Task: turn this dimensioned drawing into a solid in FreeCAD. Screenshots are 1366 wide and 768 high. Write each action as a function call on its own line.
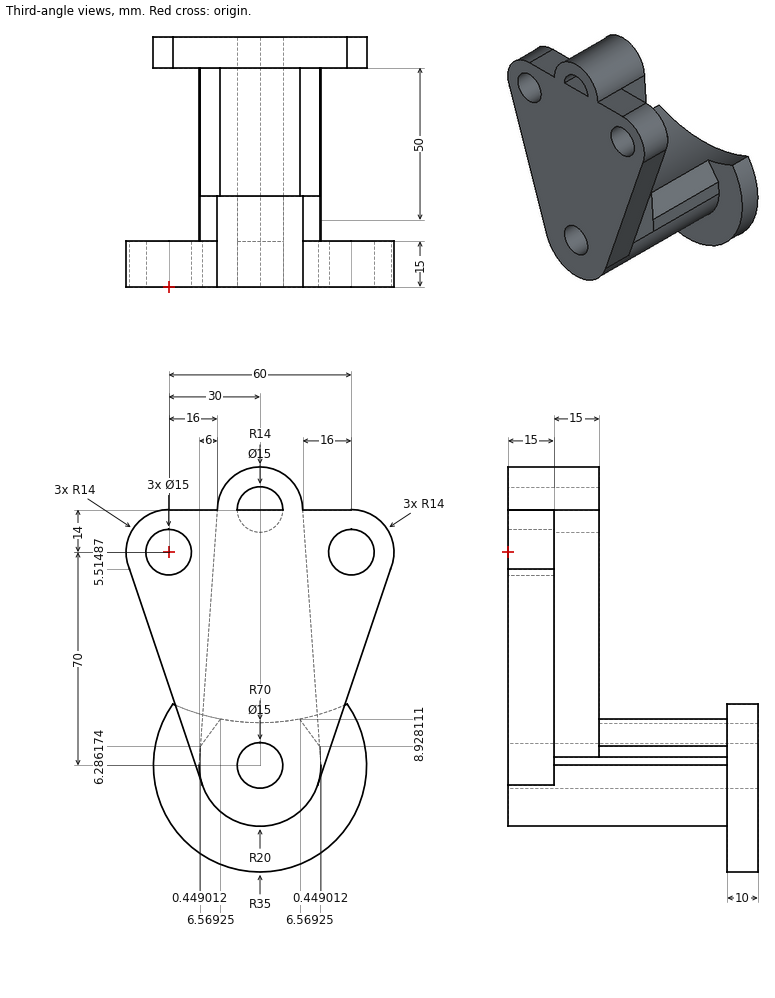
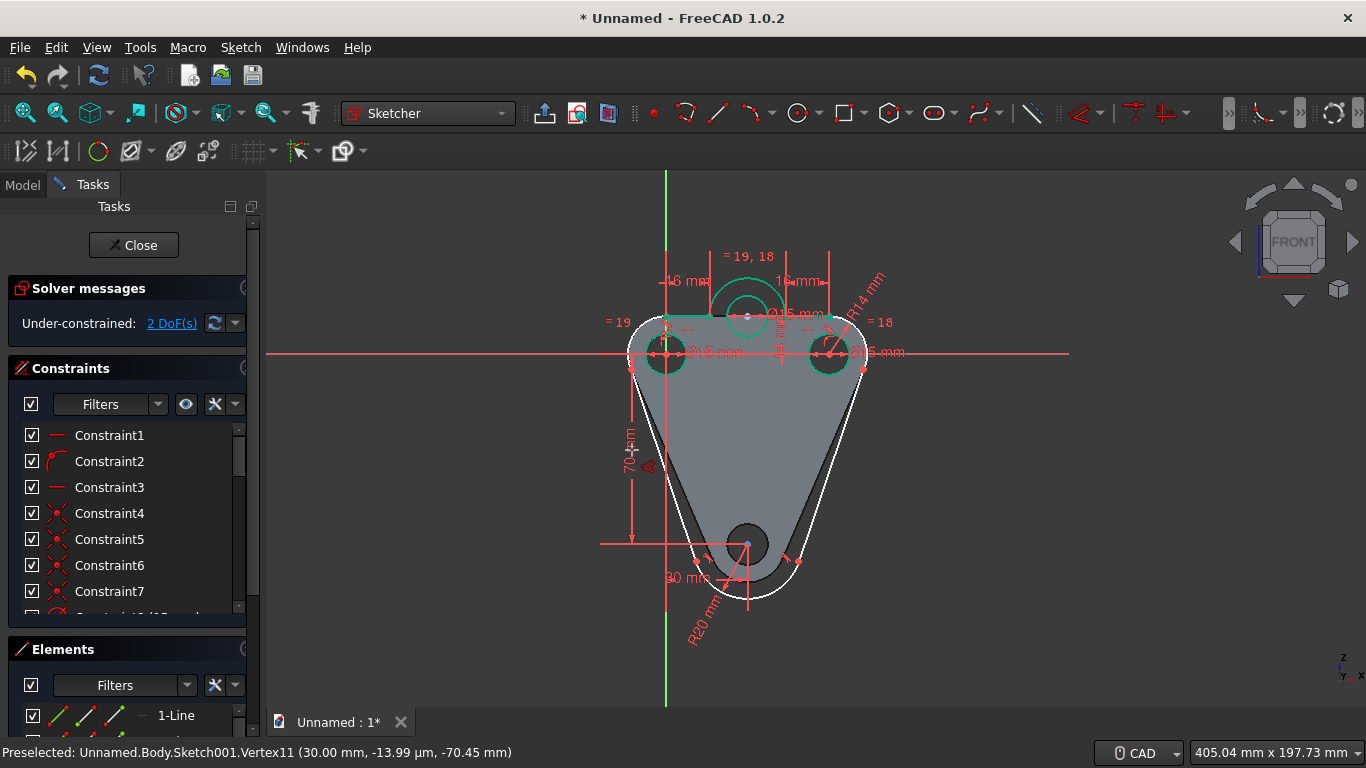
scroll(631, 370, up, 5)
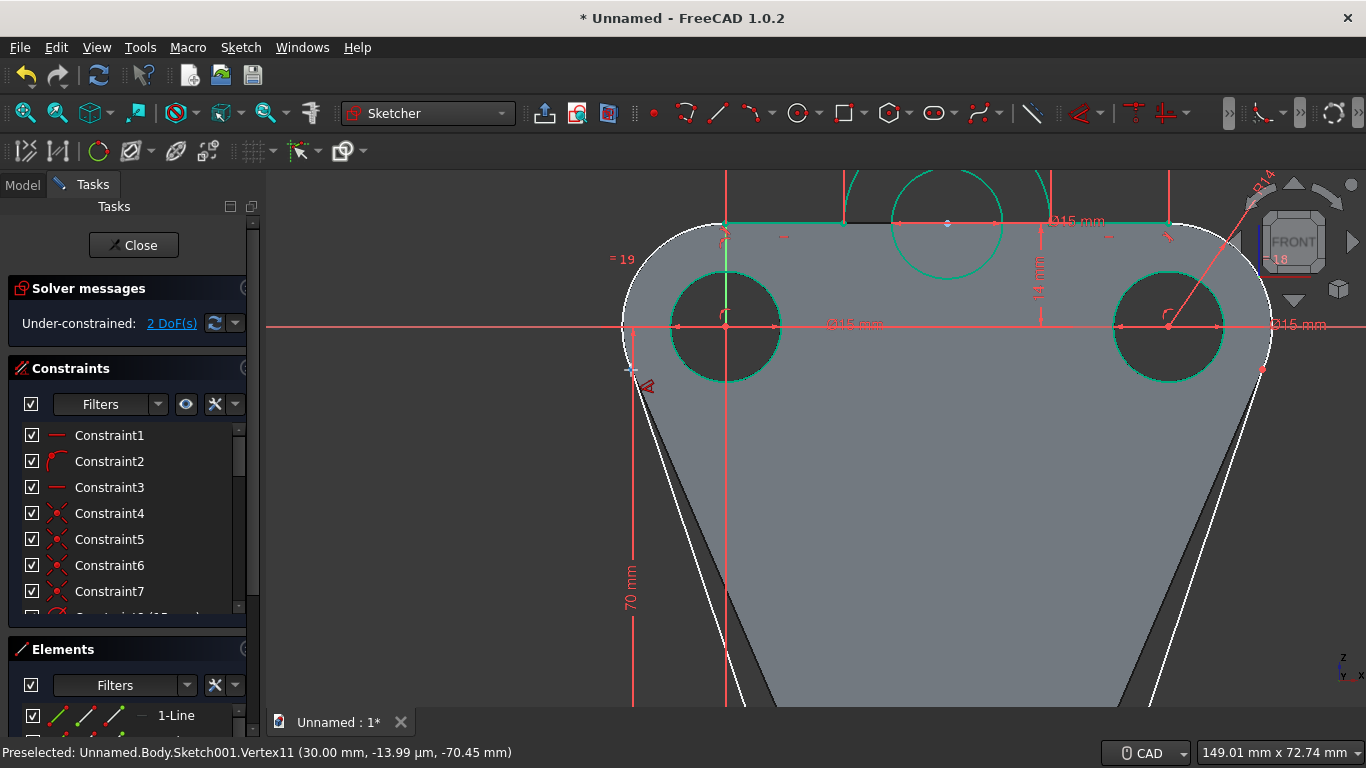
click(632, 369)
click(598, 348)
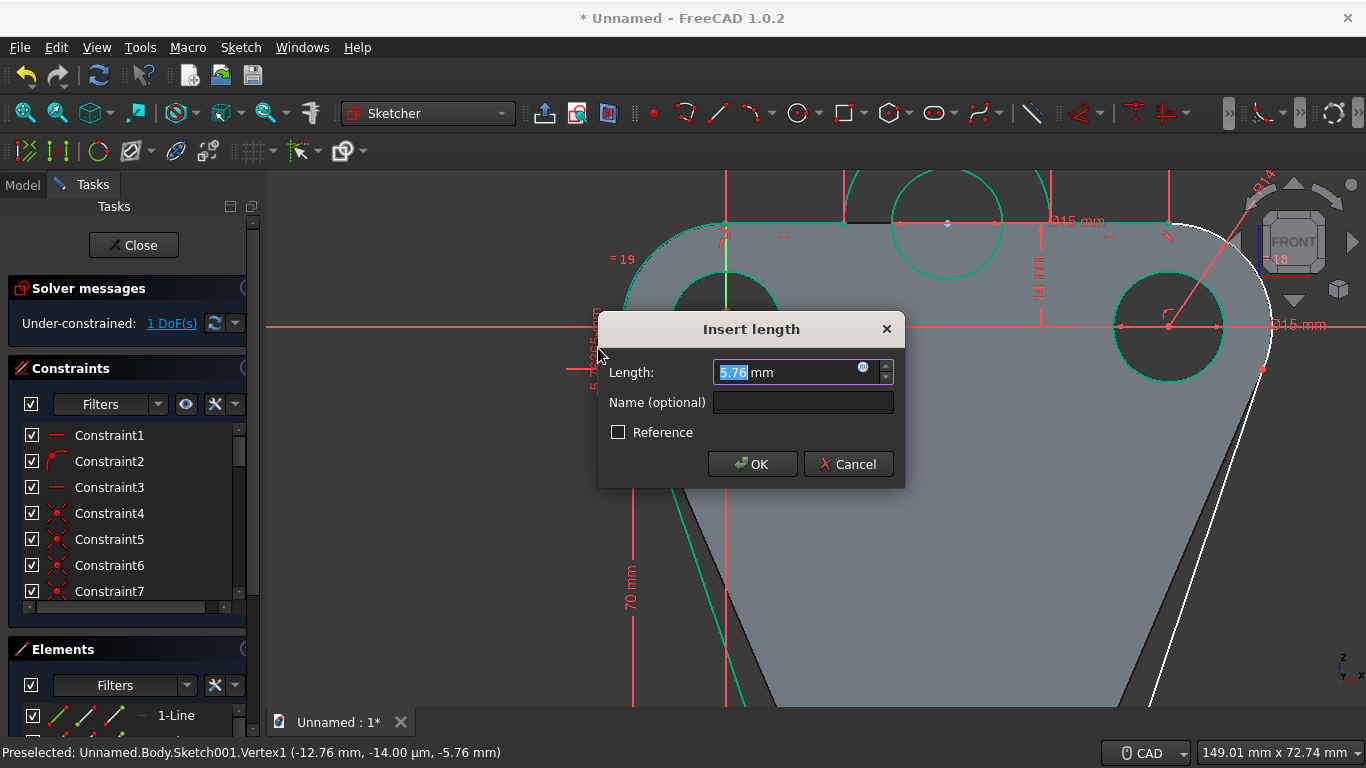
text(5.51487)
key(Return)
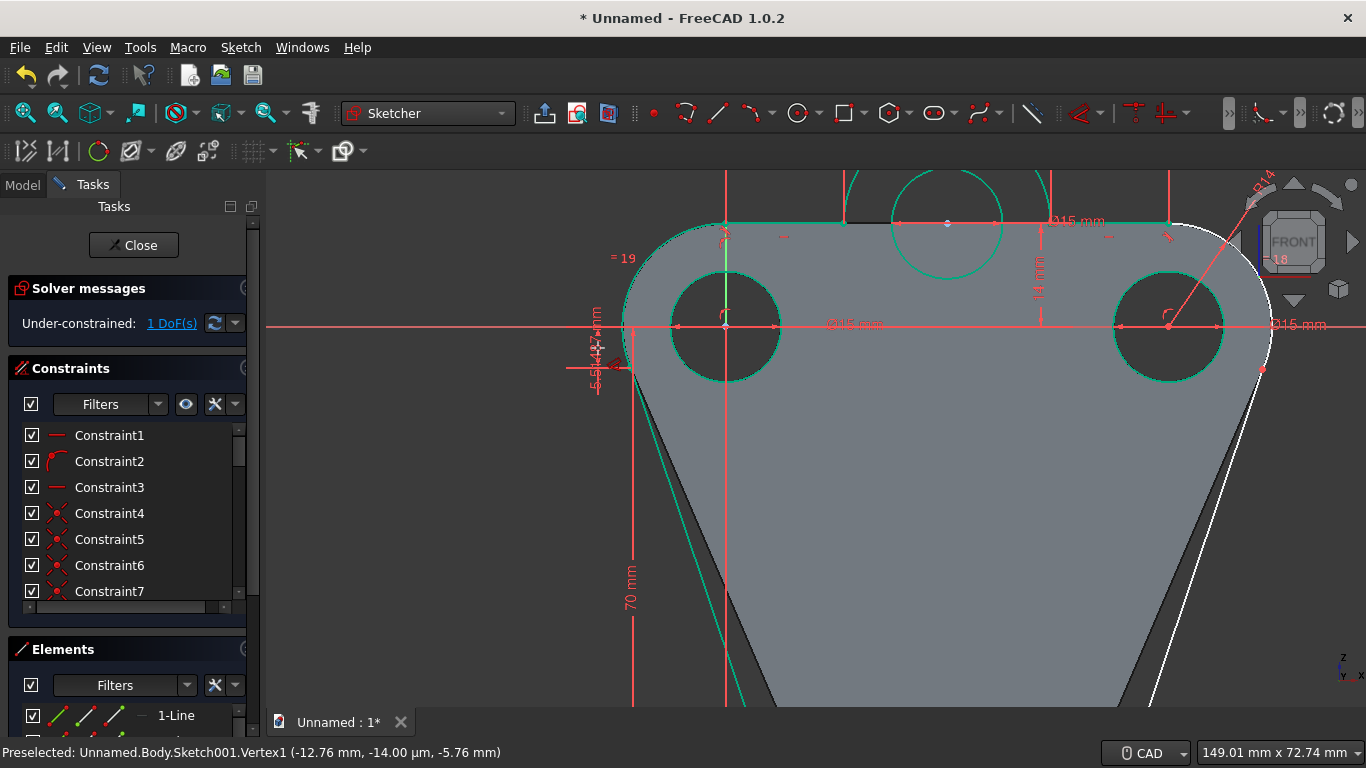
scroll(631, 370, down, 5)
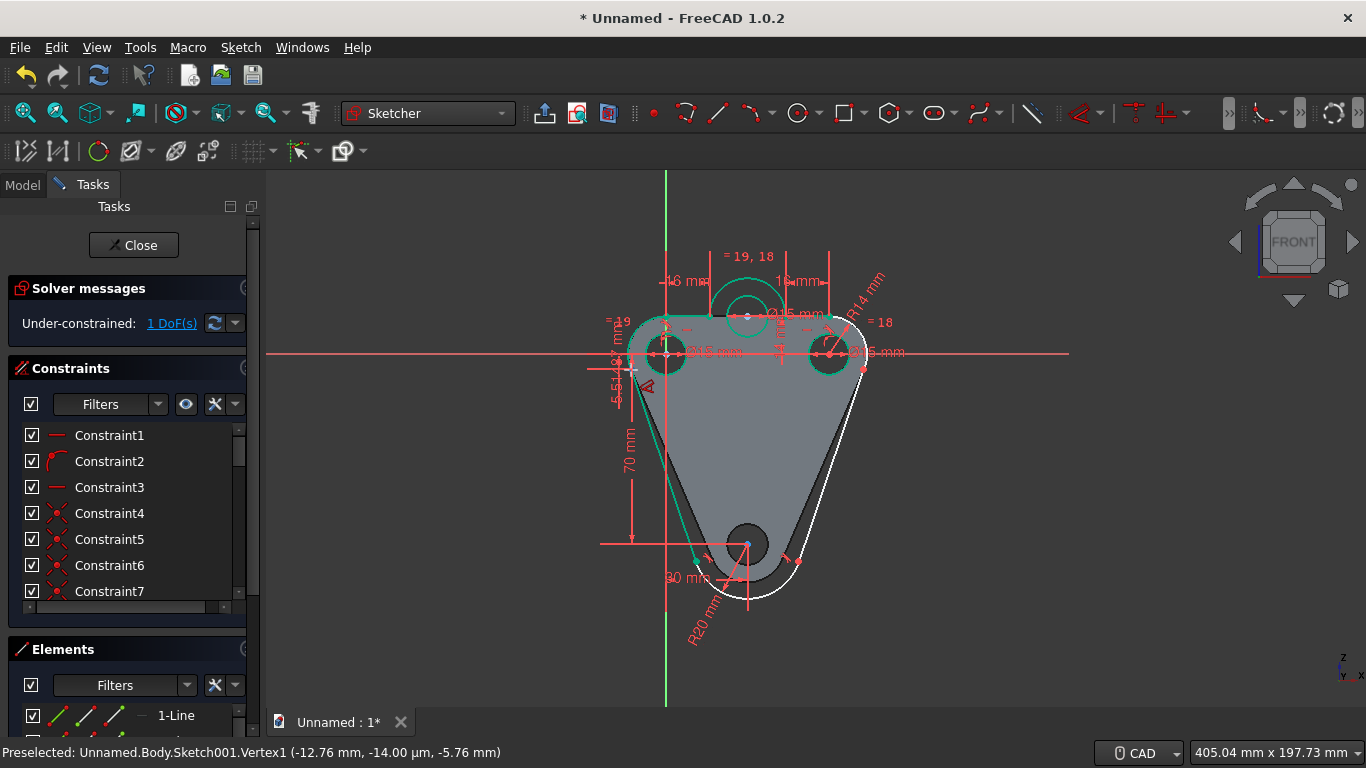
scroll(864, 370, up, 5)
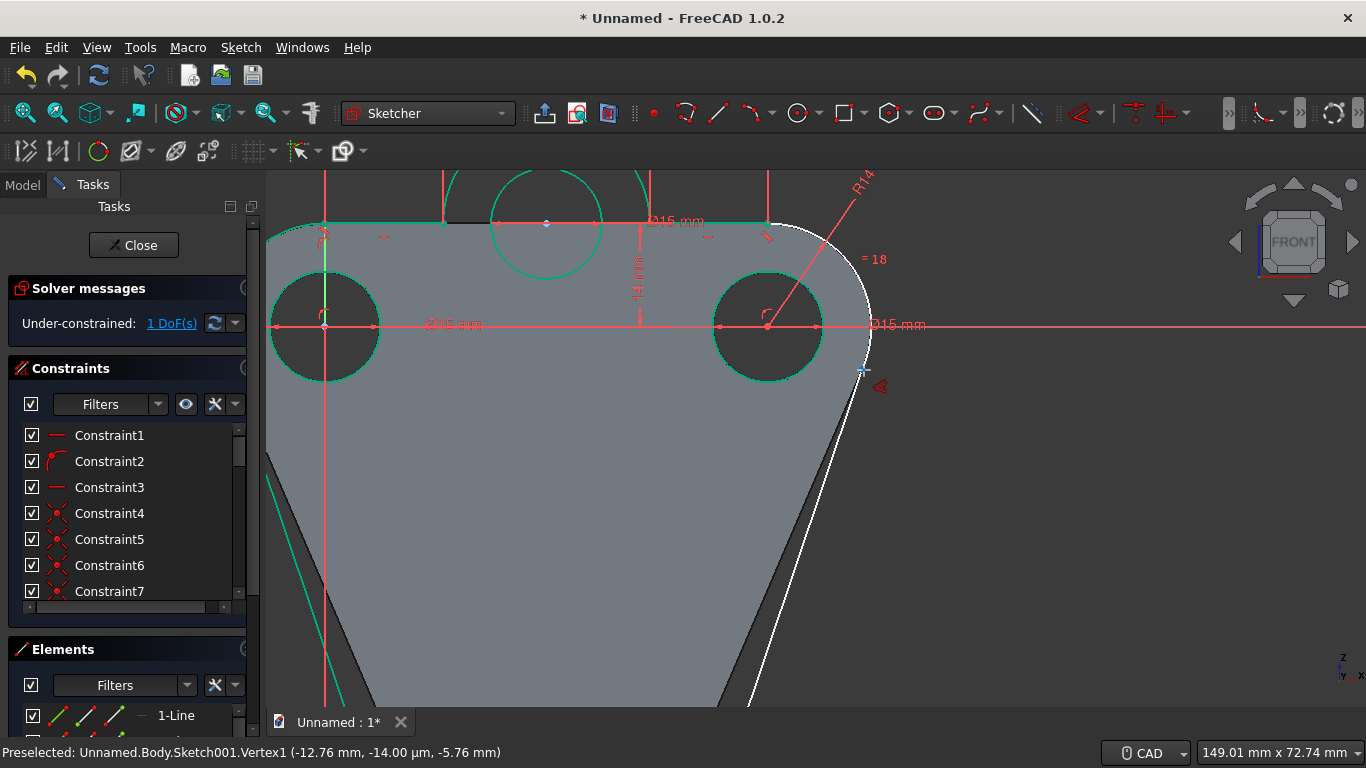
click(862, 369)
click(896, 348)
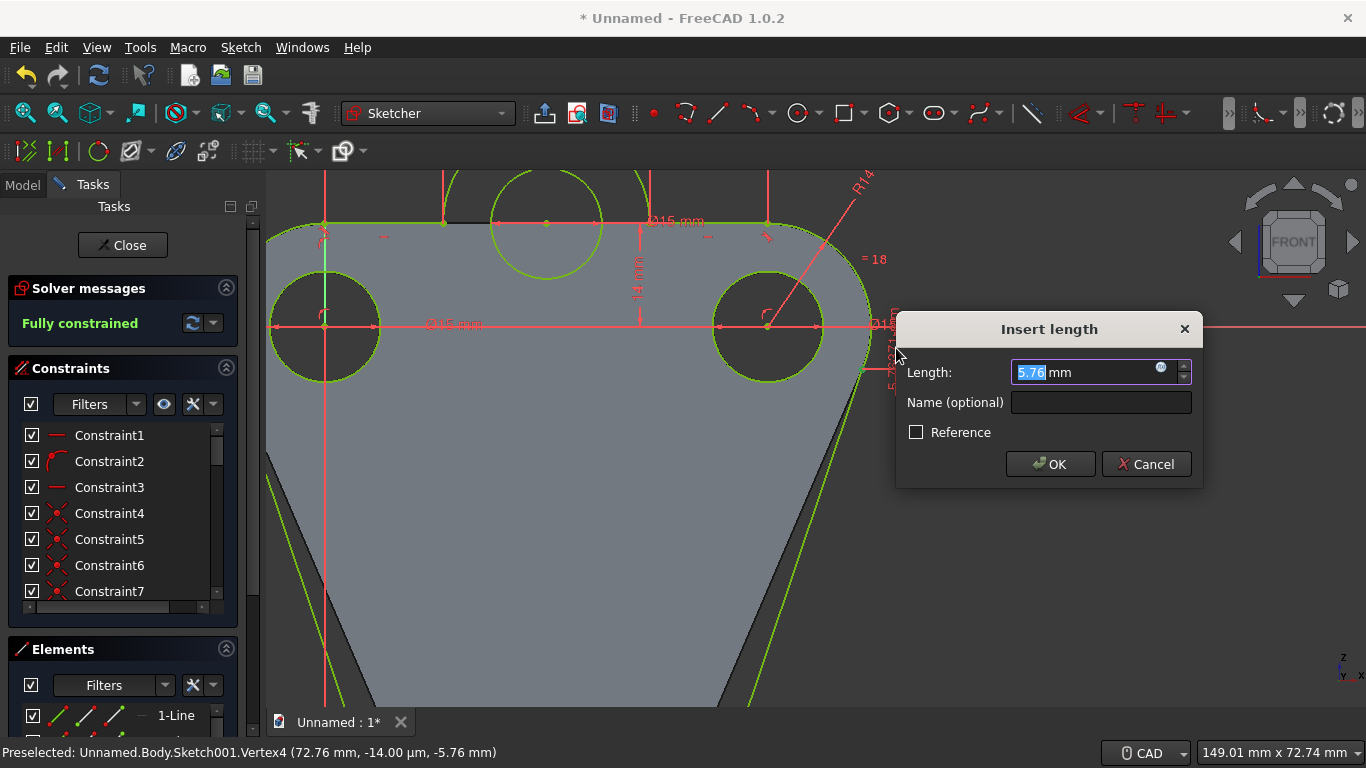
text(5.51487)
key(Return)
key(Escape)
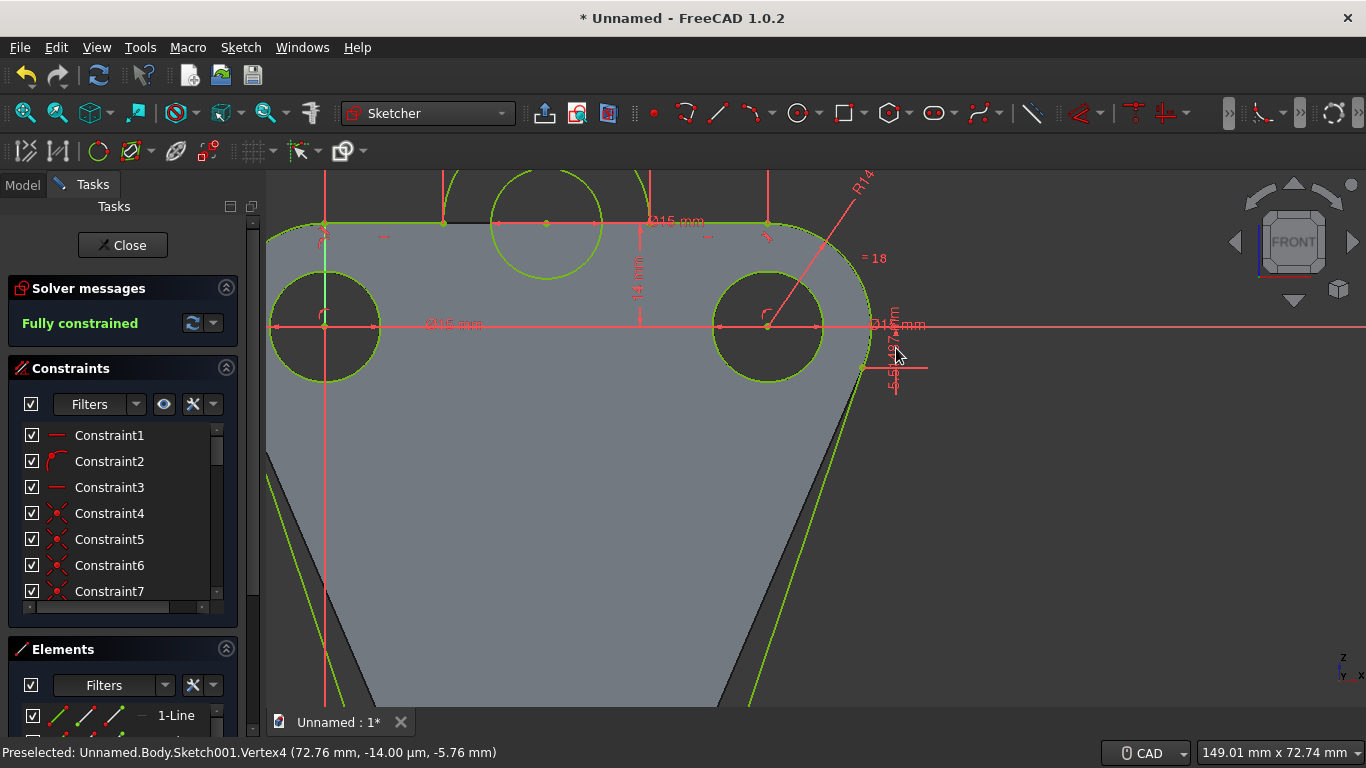
click(123, 245)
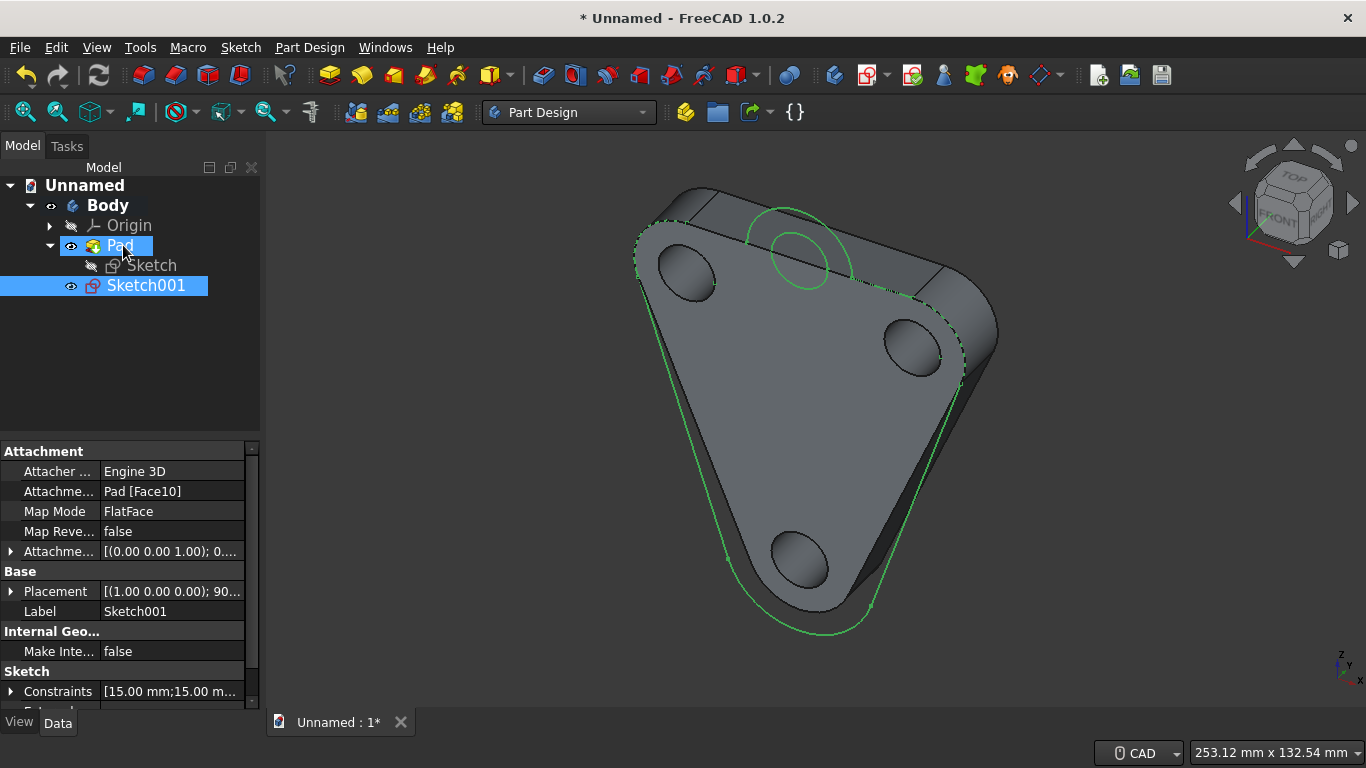
click(330, 76)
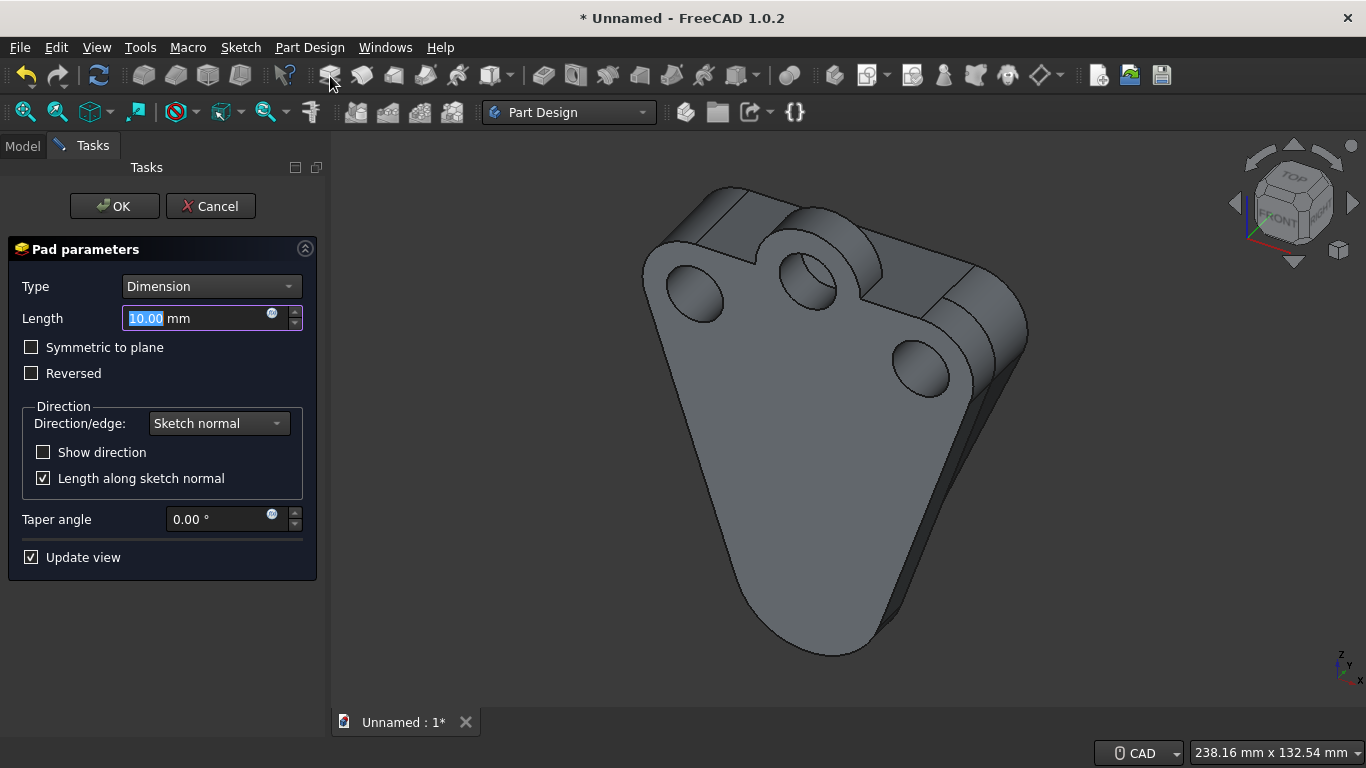
text(15)
key(Tab)